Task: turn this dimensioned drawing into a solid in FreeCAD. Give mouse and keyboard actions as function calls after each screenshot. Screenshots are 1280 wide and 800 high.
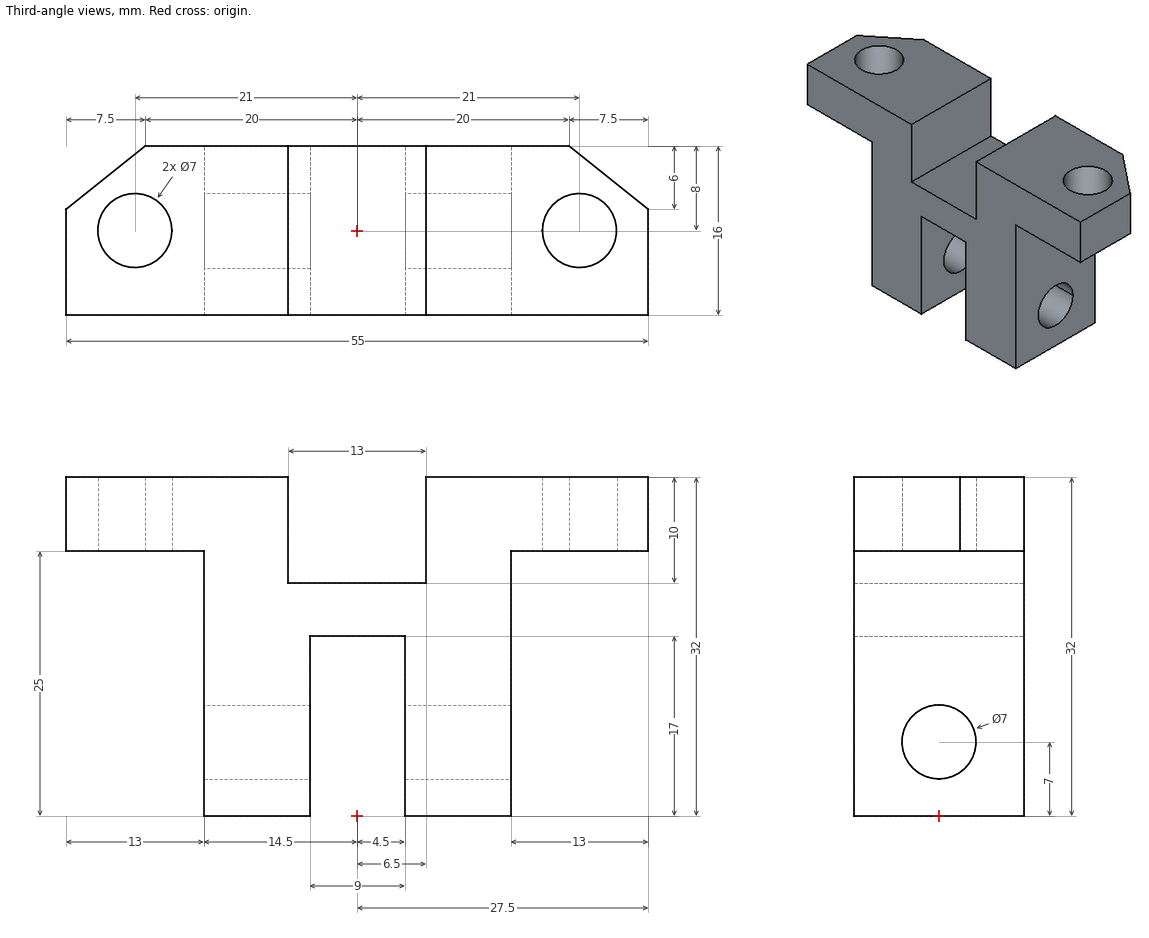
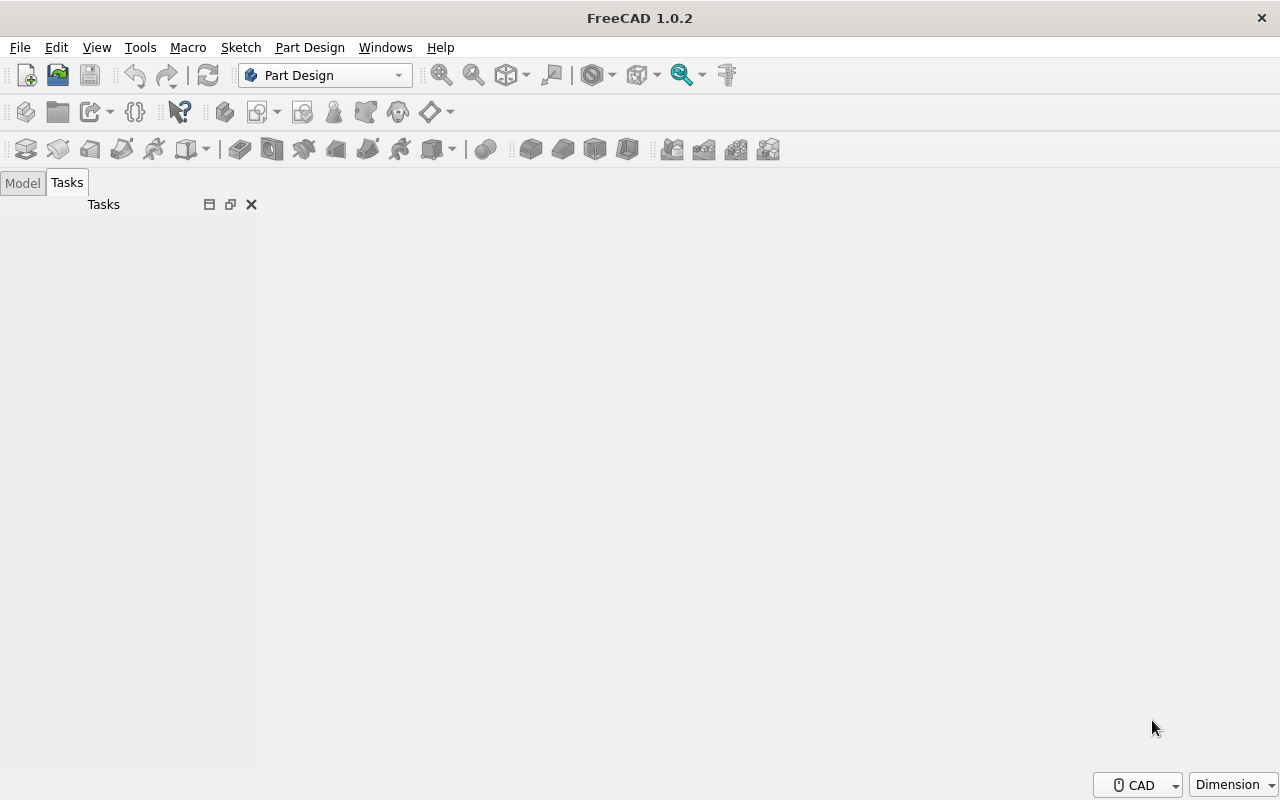
click(26, 76)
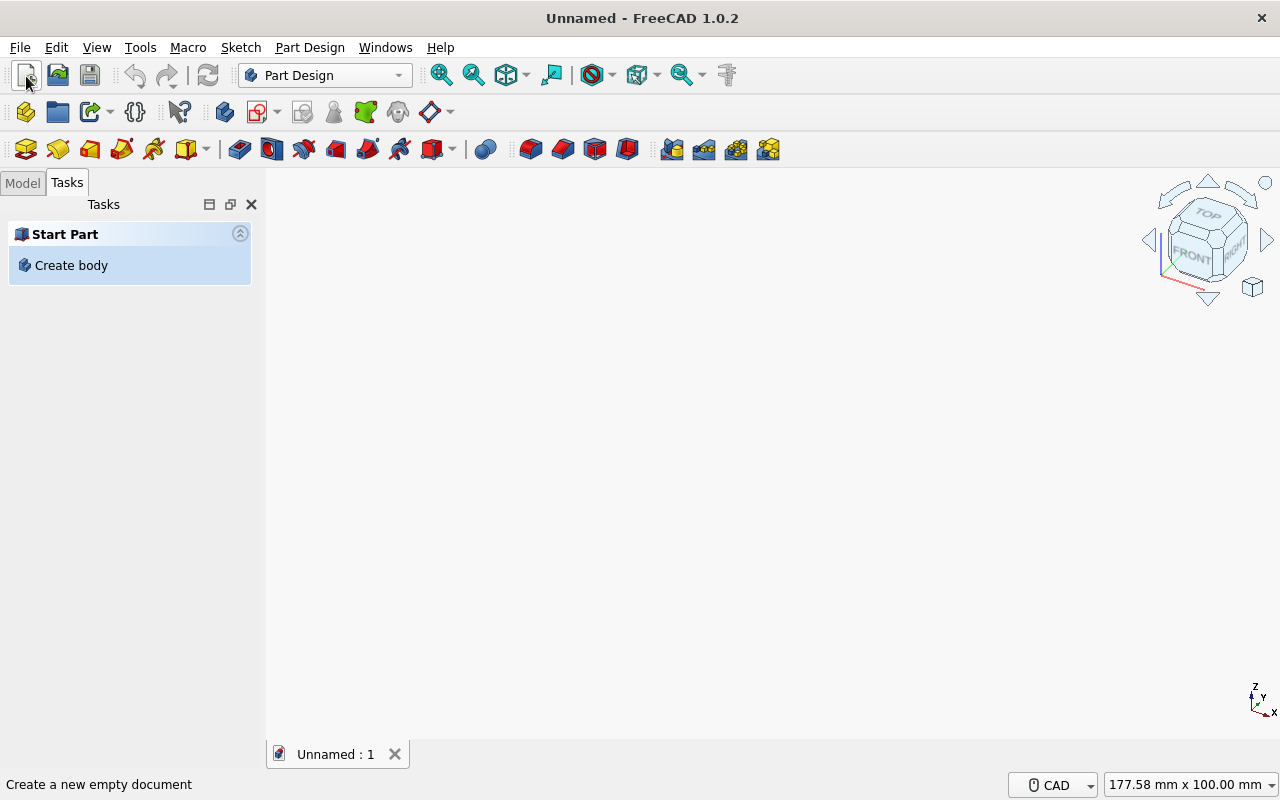
click(258, 112)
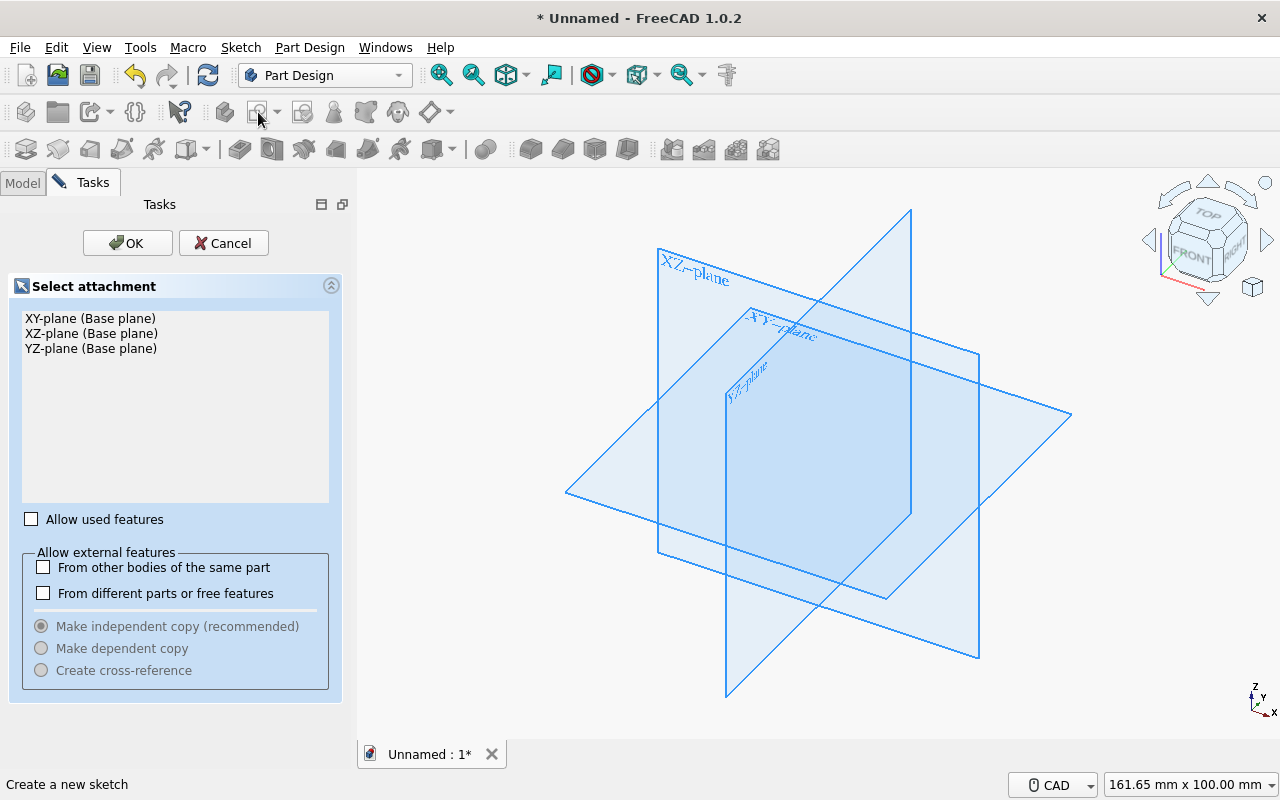
click(82, 318)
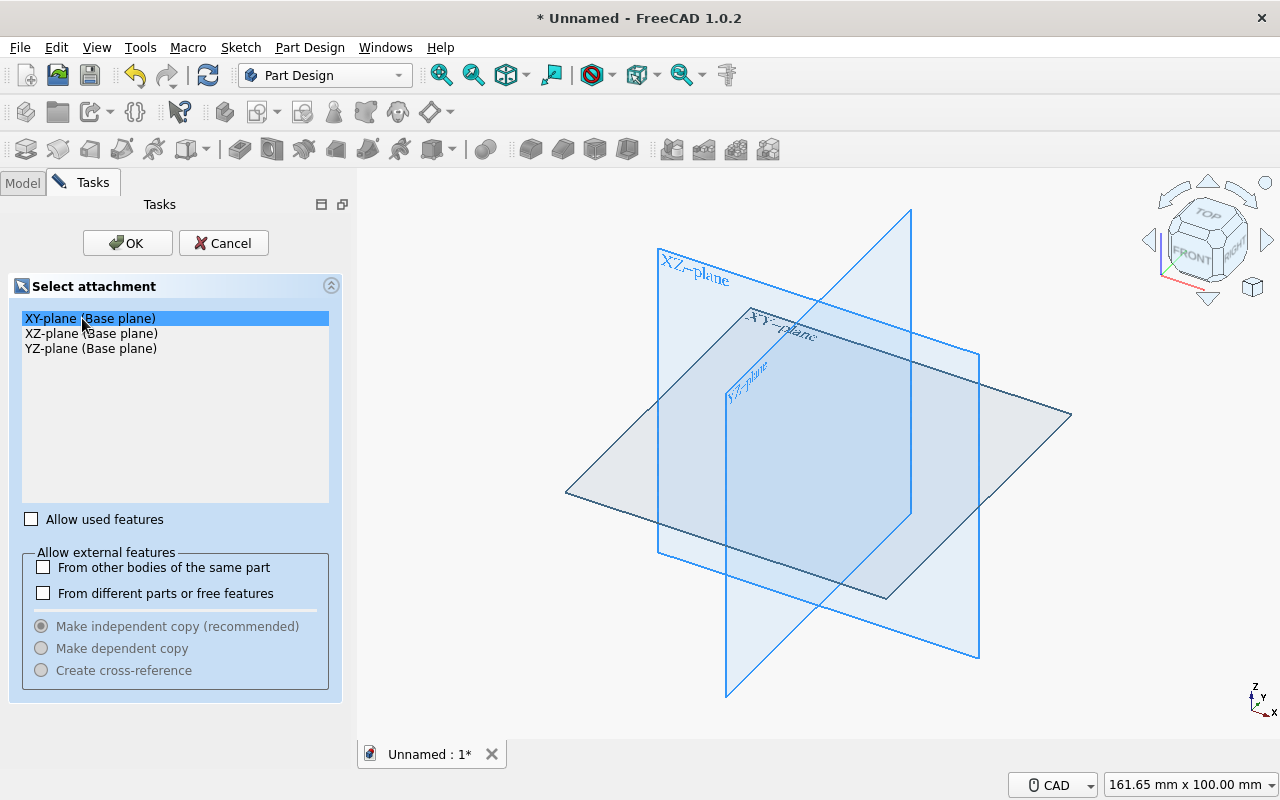
click(128, 243)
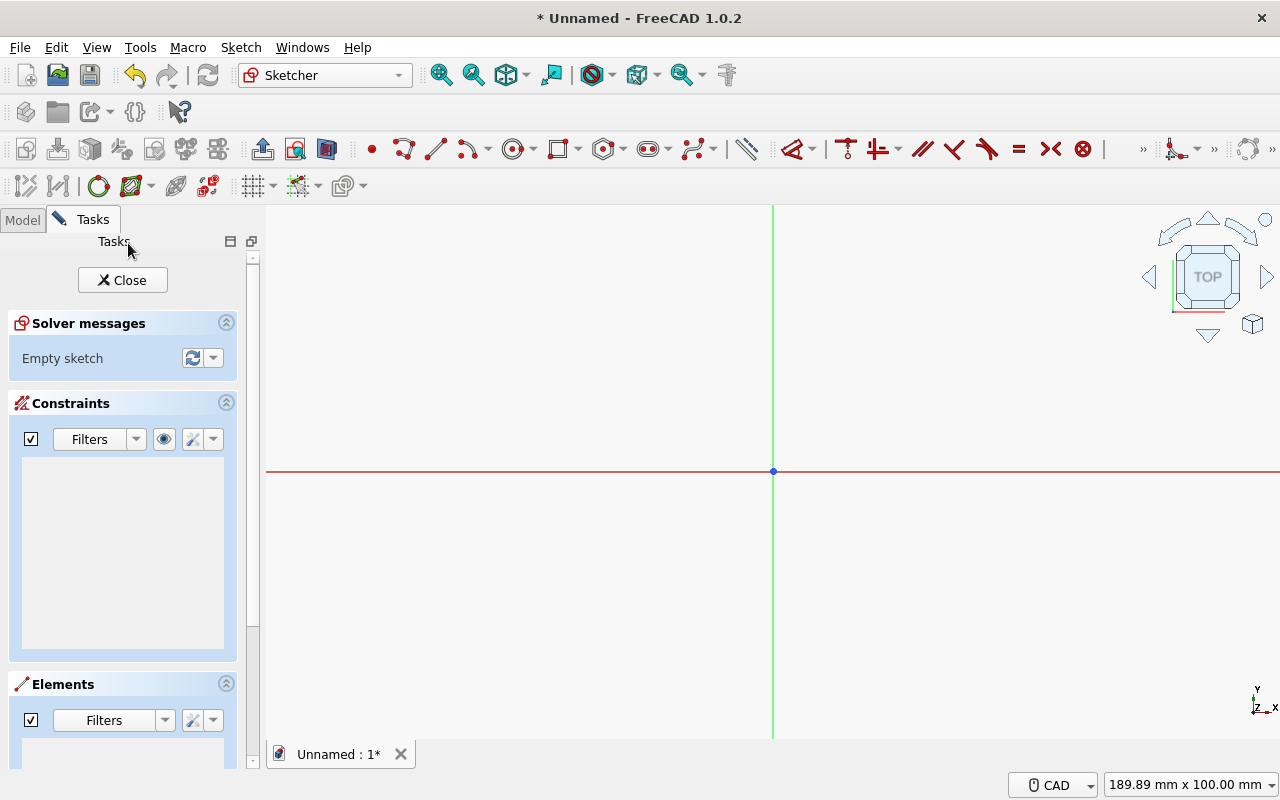
scroll(856, 472, up, 3)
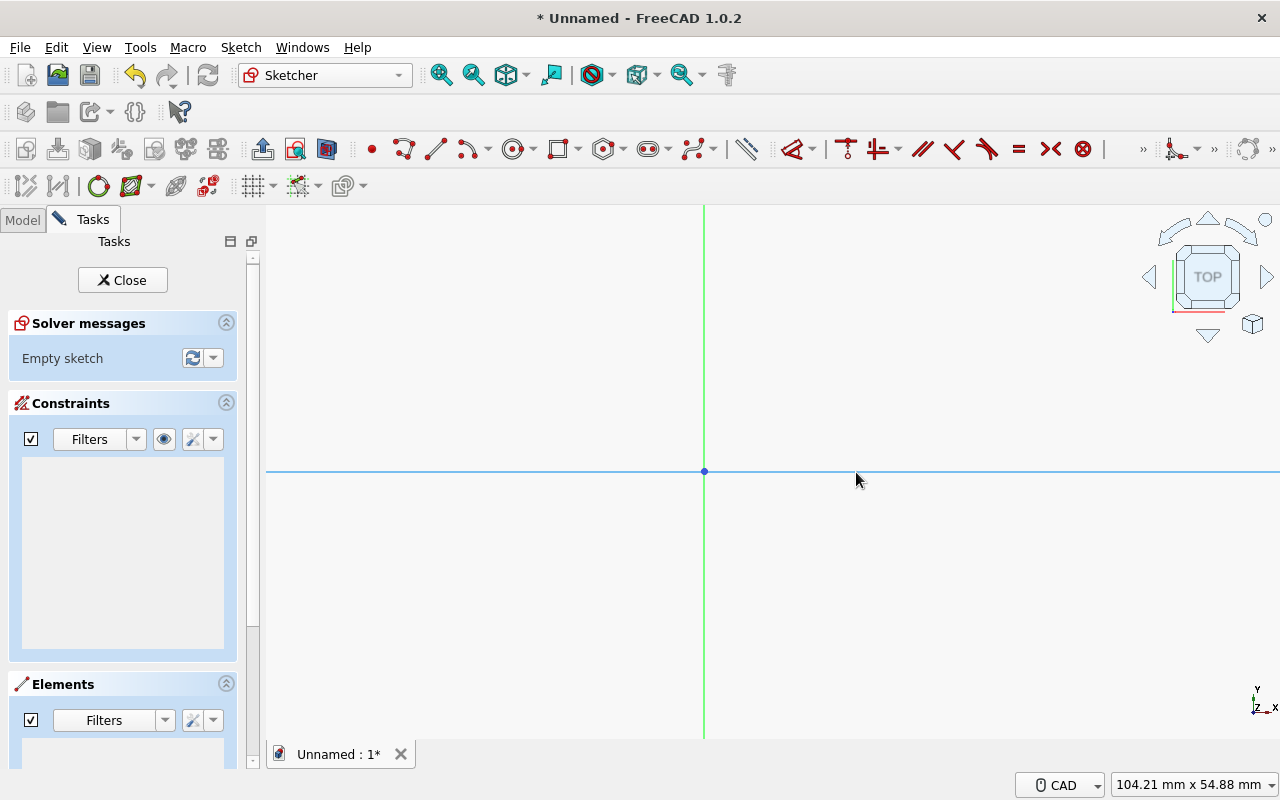
key(g)
key(v)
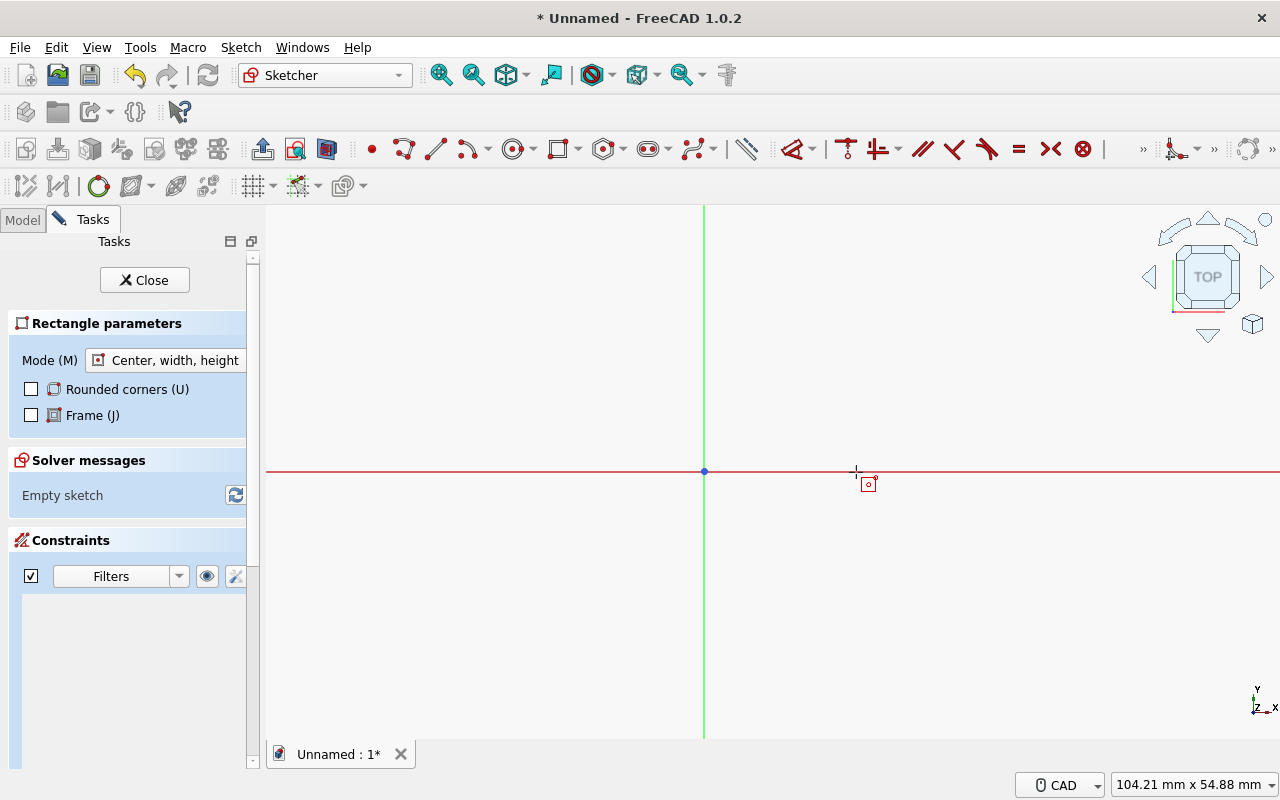
click(704, 472)
click(972, 394)
key(Escape)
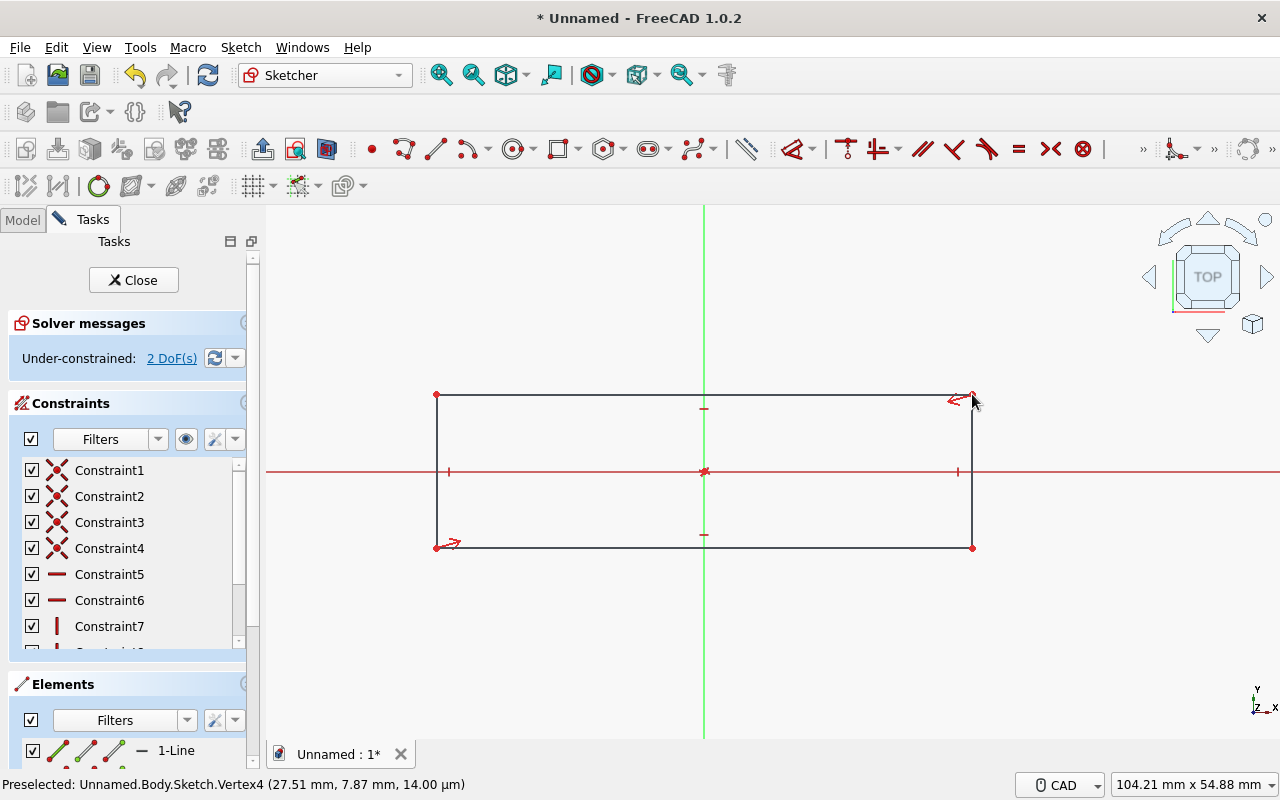
click(597, 548)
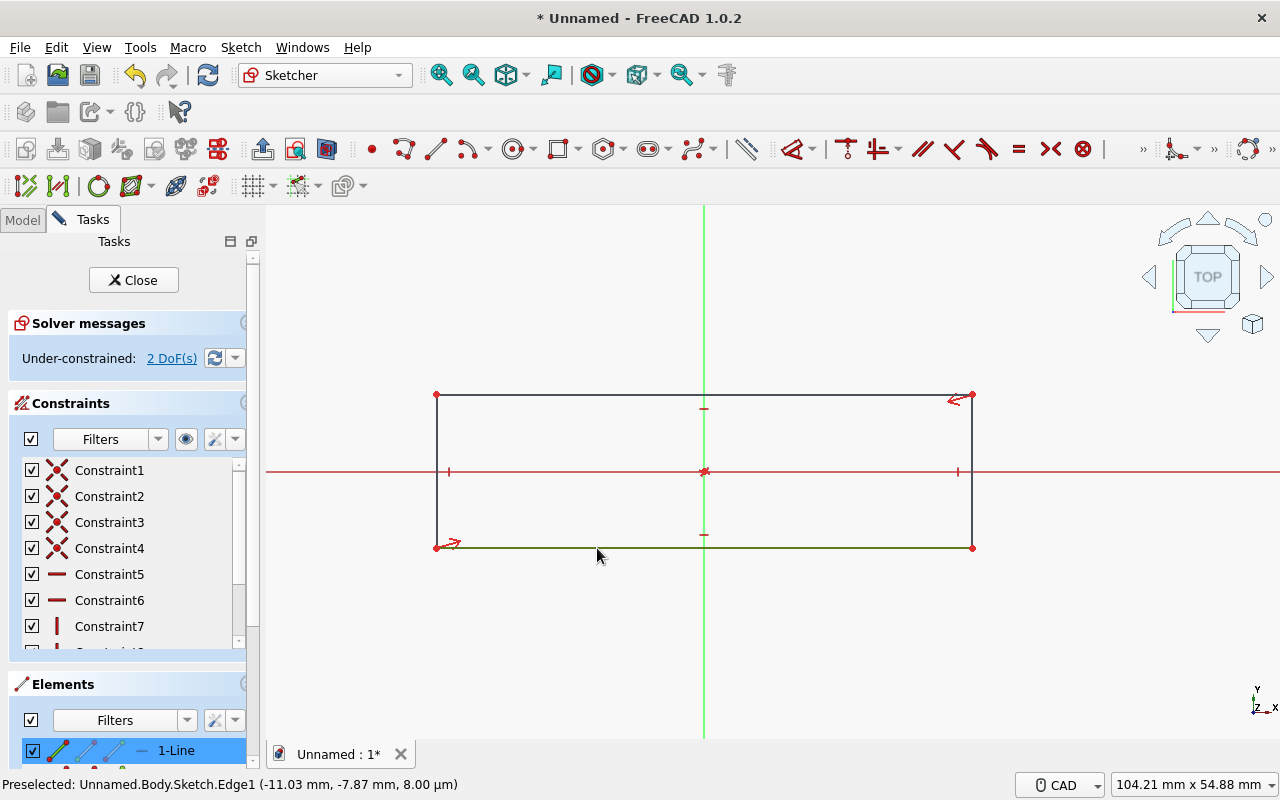
click(814, 150)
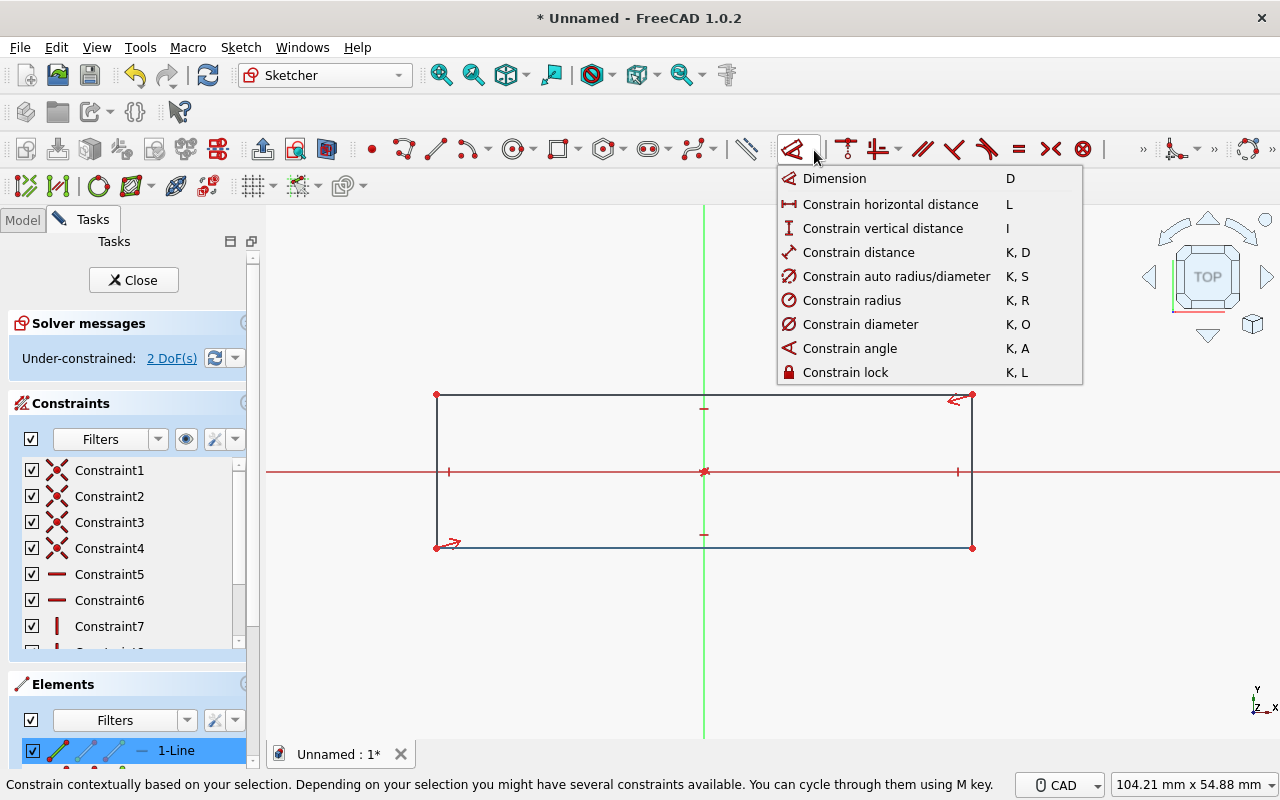
click(930, 204)